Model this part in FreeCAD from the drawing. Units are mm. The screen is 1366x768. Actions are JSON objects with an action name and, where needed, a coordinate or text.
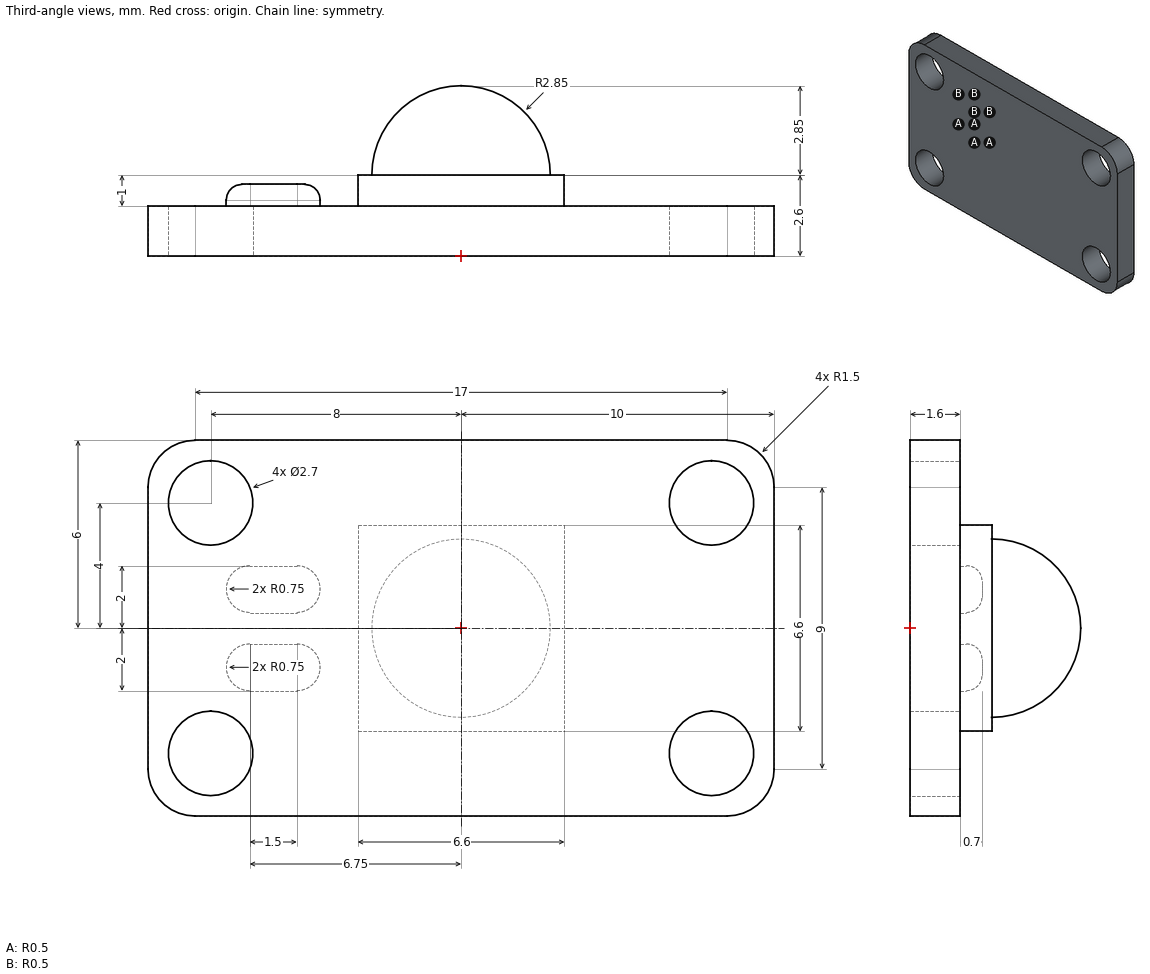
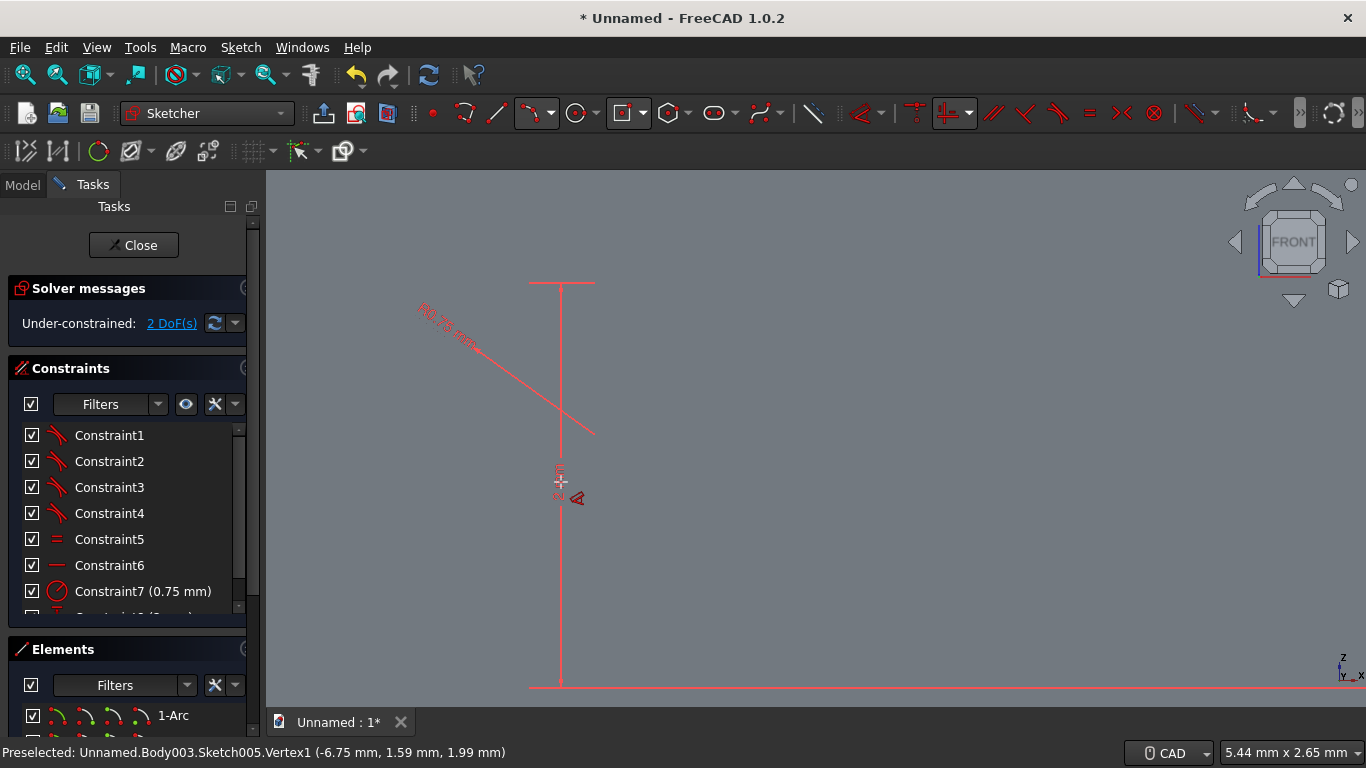
{"action": "left_click", "coordinate": [686, 283]}
{"action": "left_click", "coordinate": [746, 249]}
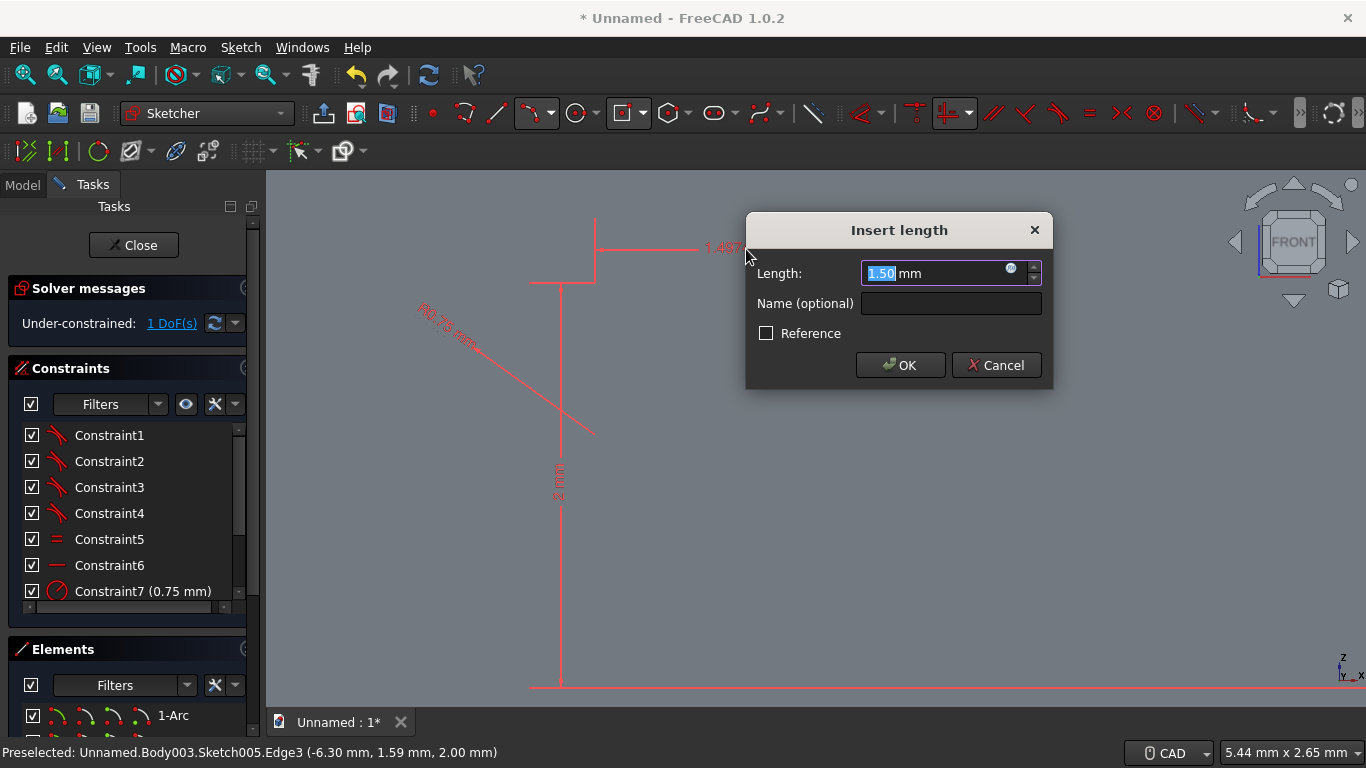
{"action": "type", "text": "1.5"}
{"action": "key", "text": "Return"}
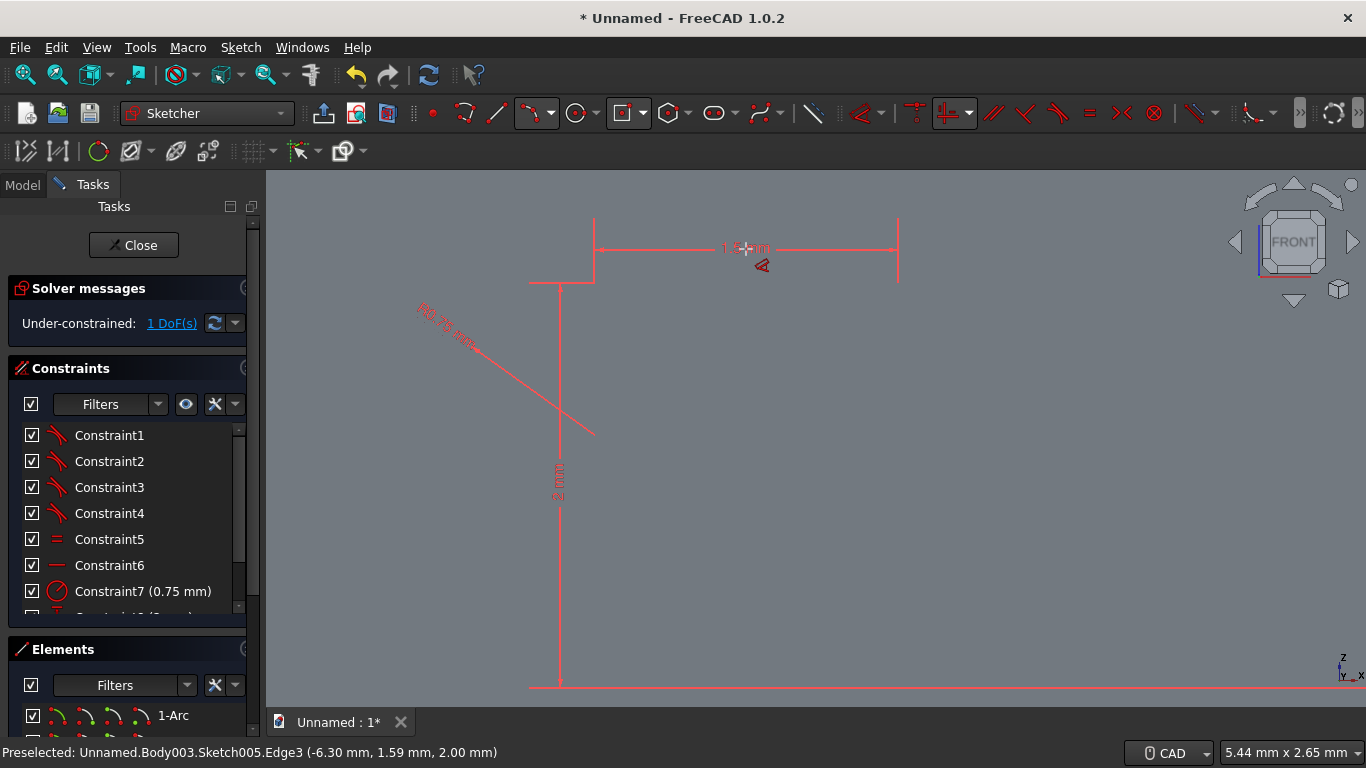
{"action": "left_click", "coordinate": [594, 283]}
{"action": "left_click", "coordinate": [898, 249]}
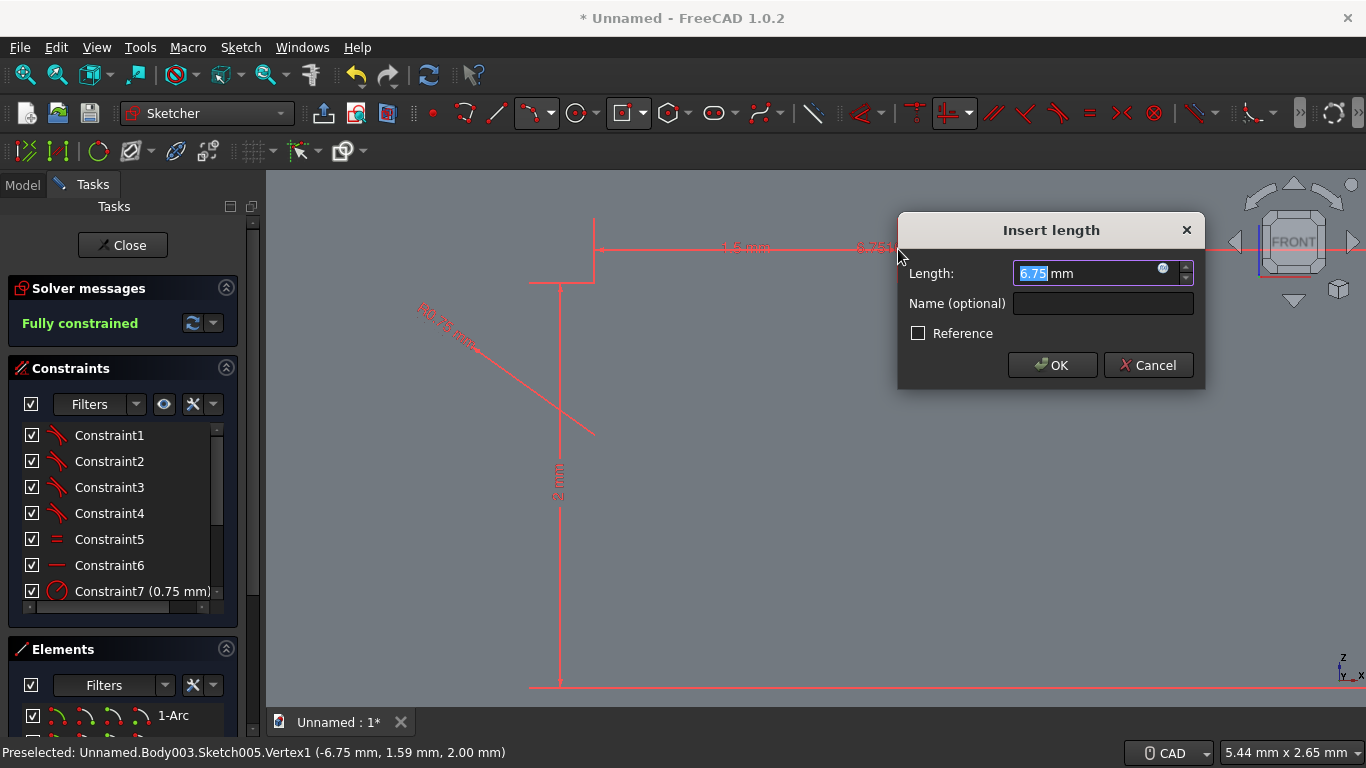
{"action": "type", "text": "6.75"}
{"action": "key", "text": "Return"}
{"action": "key", "text": "Escape"}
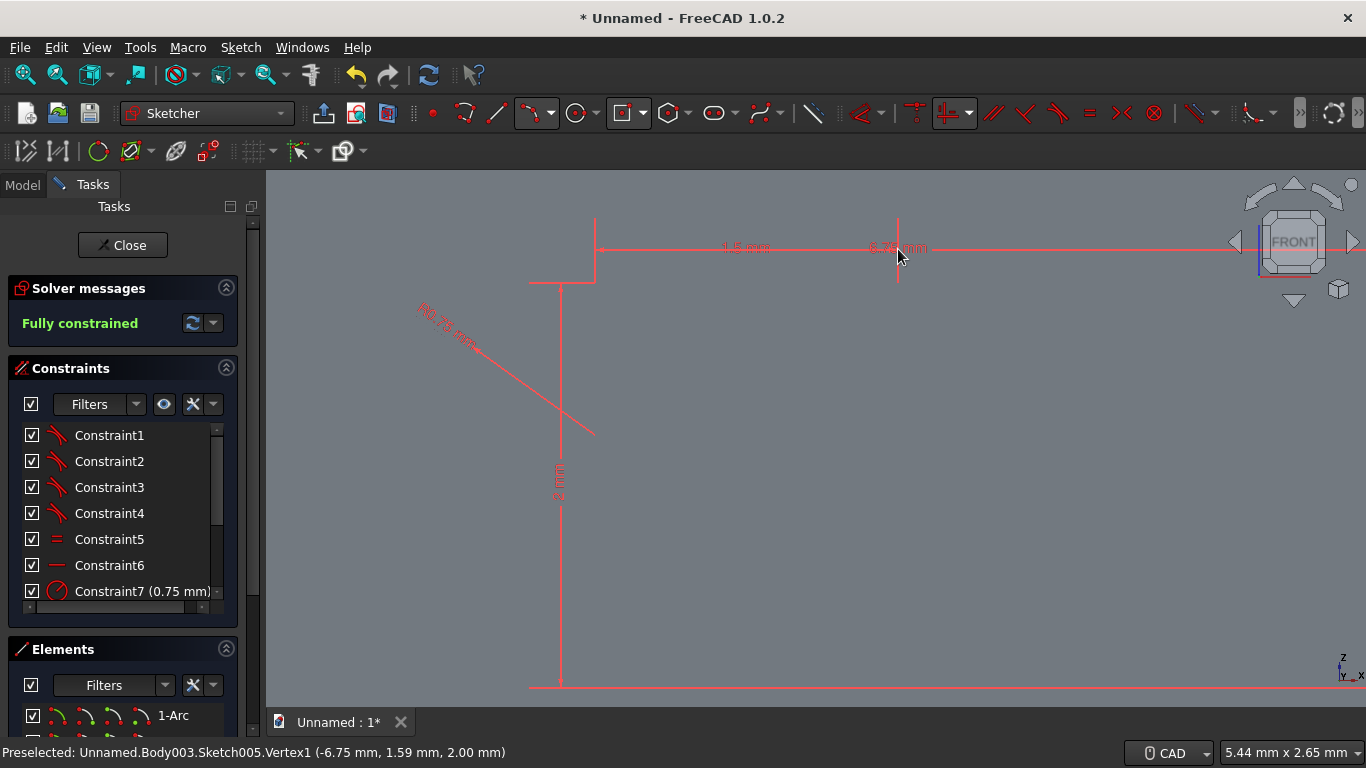
{"action": "left_click", "coordinate": [123, 245]}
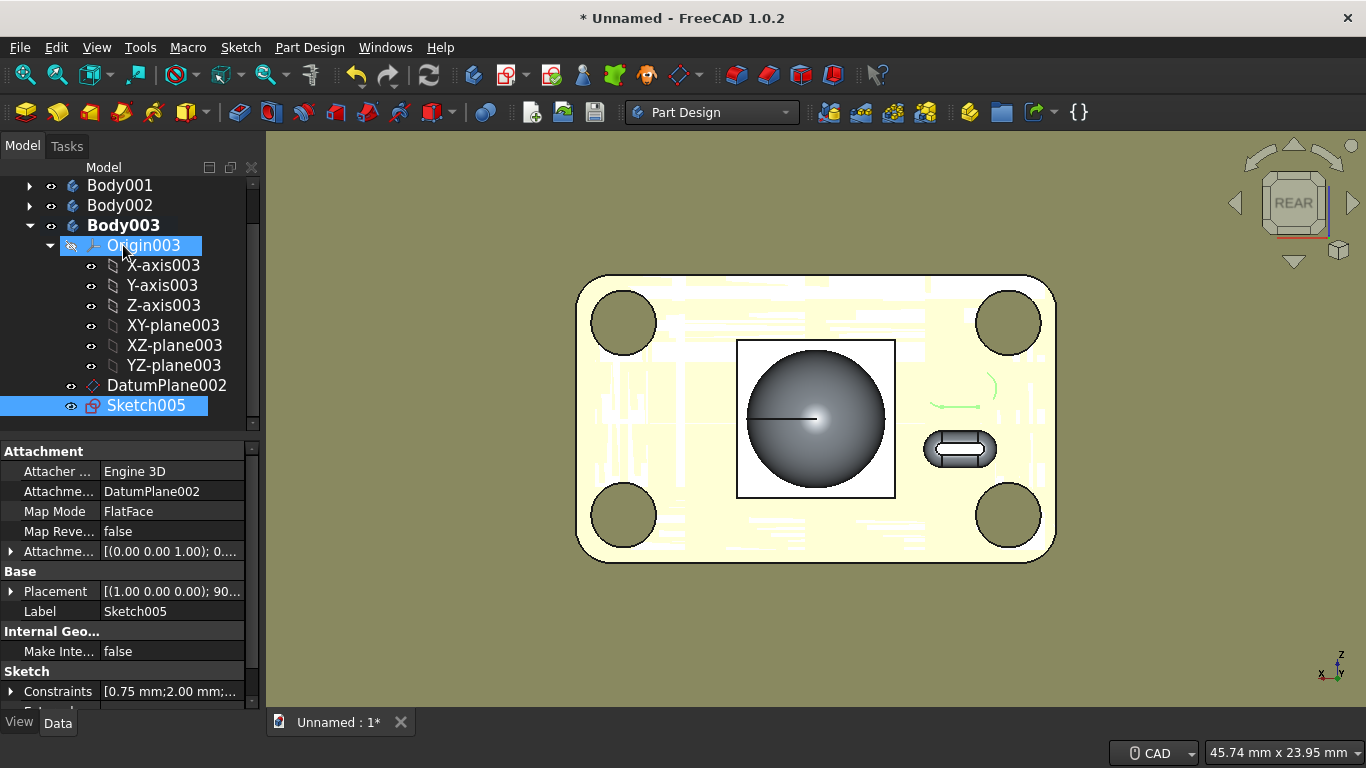
{"action": "left_click", "coordinate": [26, 112]}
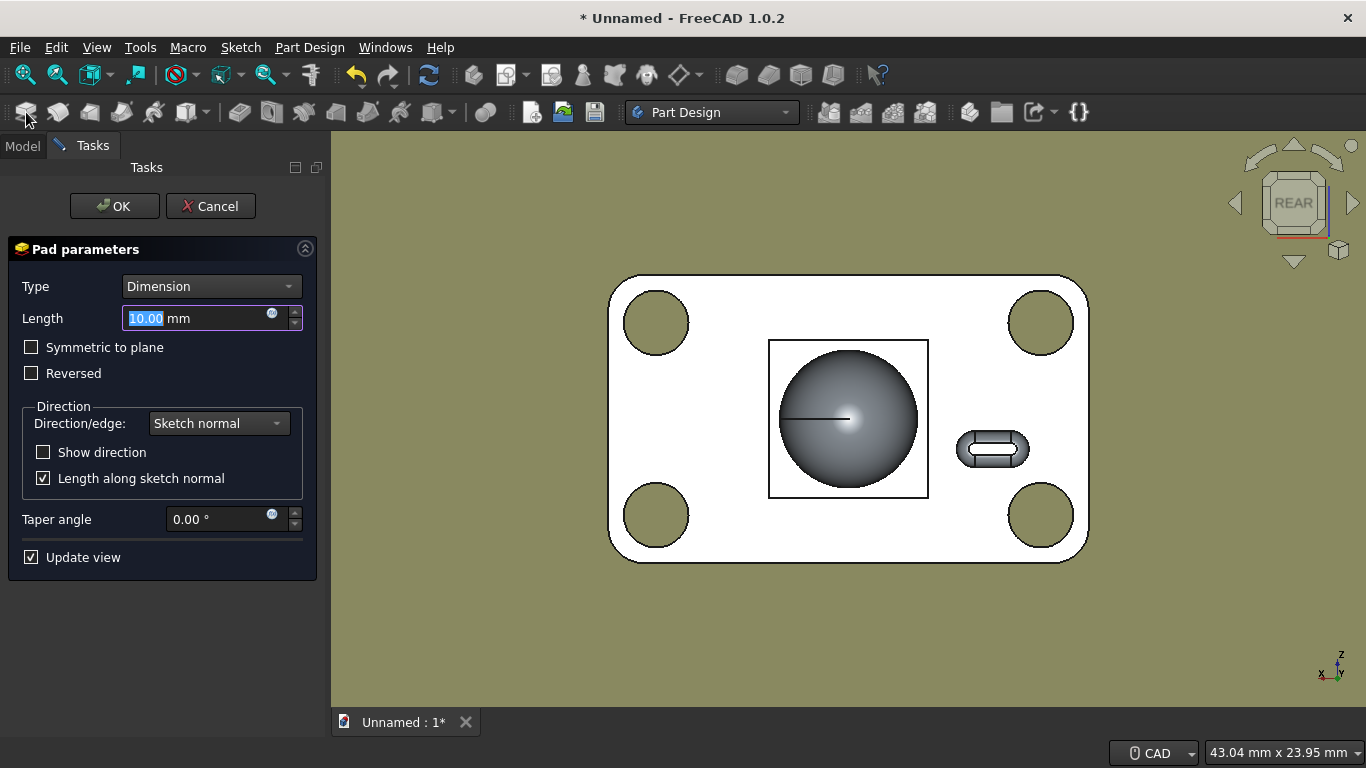
{"action": "type", "text": "0.7"}
{"action": "key", "text": "Tab"}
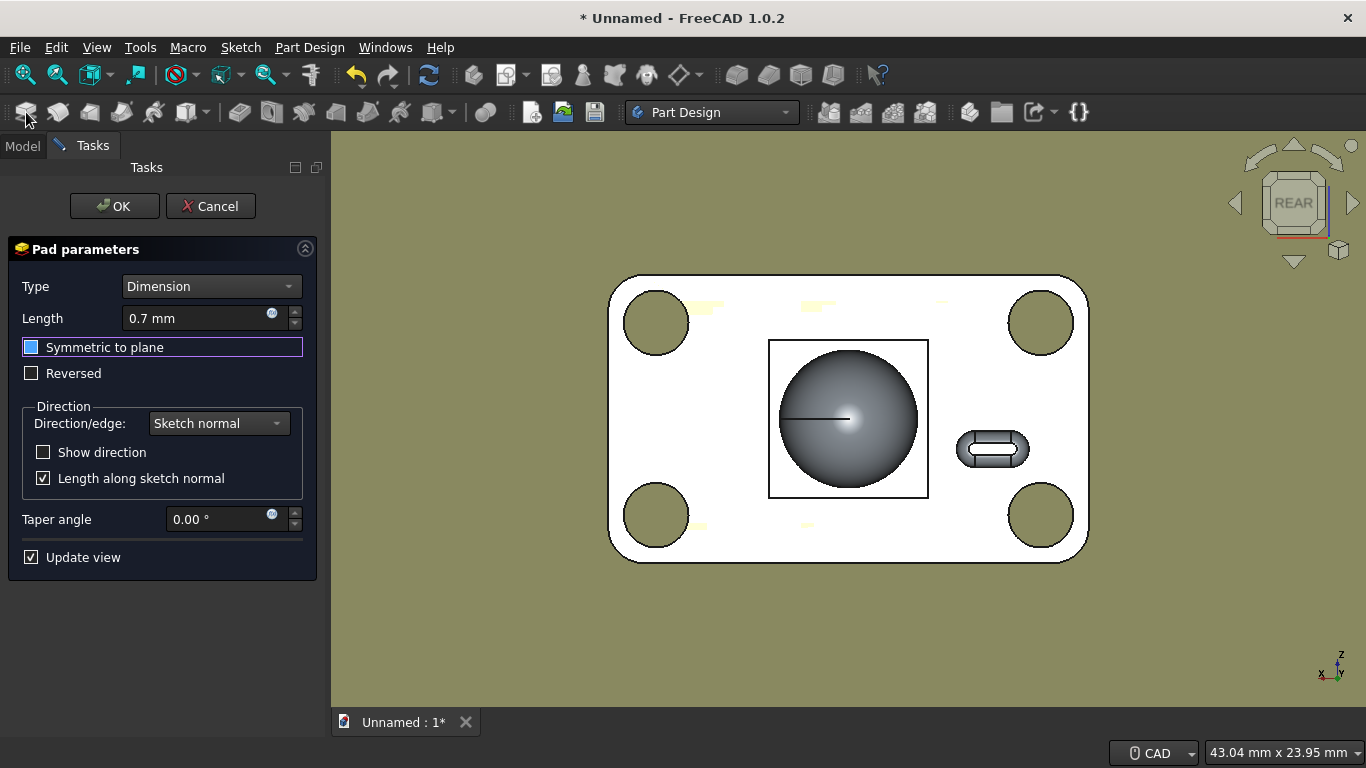
{"action": "left_click", "coordinate": [30, 373]}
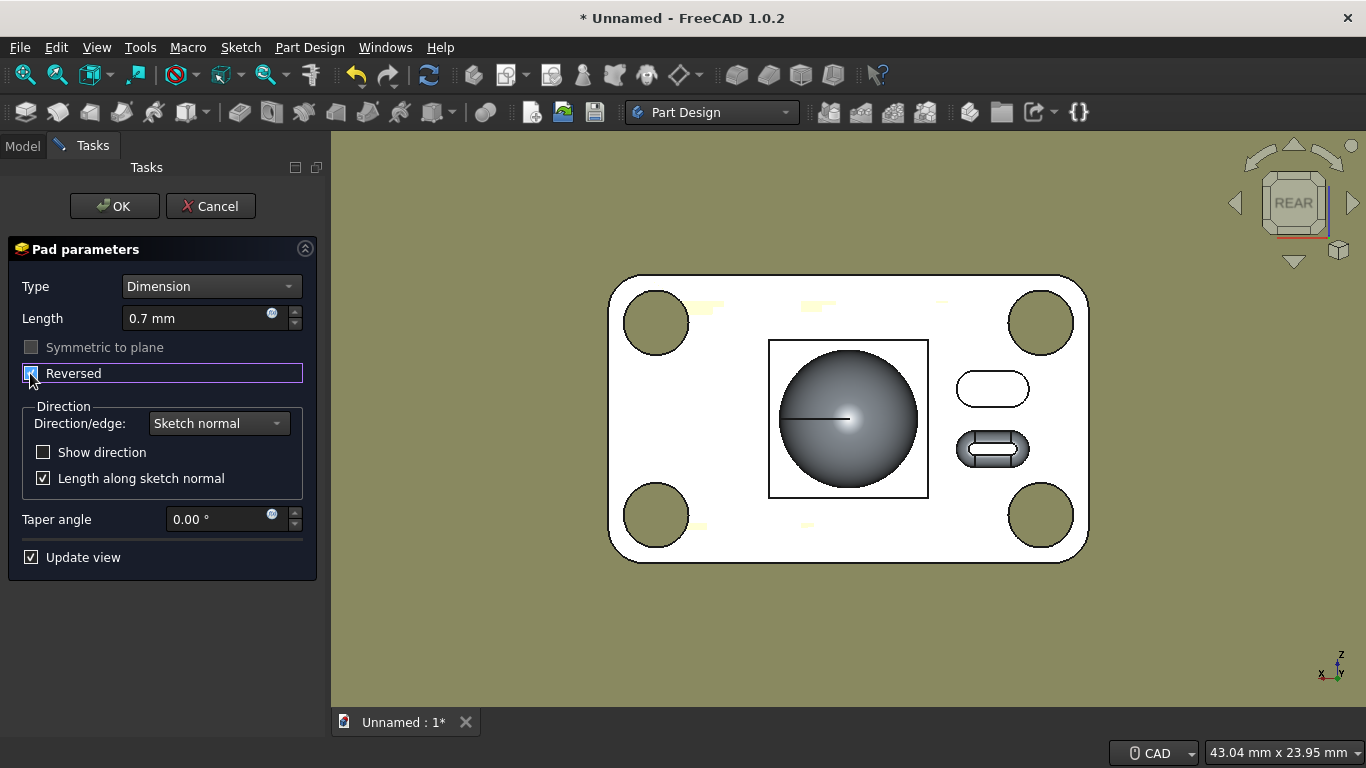
{"action": "left_click", "coordinate": [115, 206]}